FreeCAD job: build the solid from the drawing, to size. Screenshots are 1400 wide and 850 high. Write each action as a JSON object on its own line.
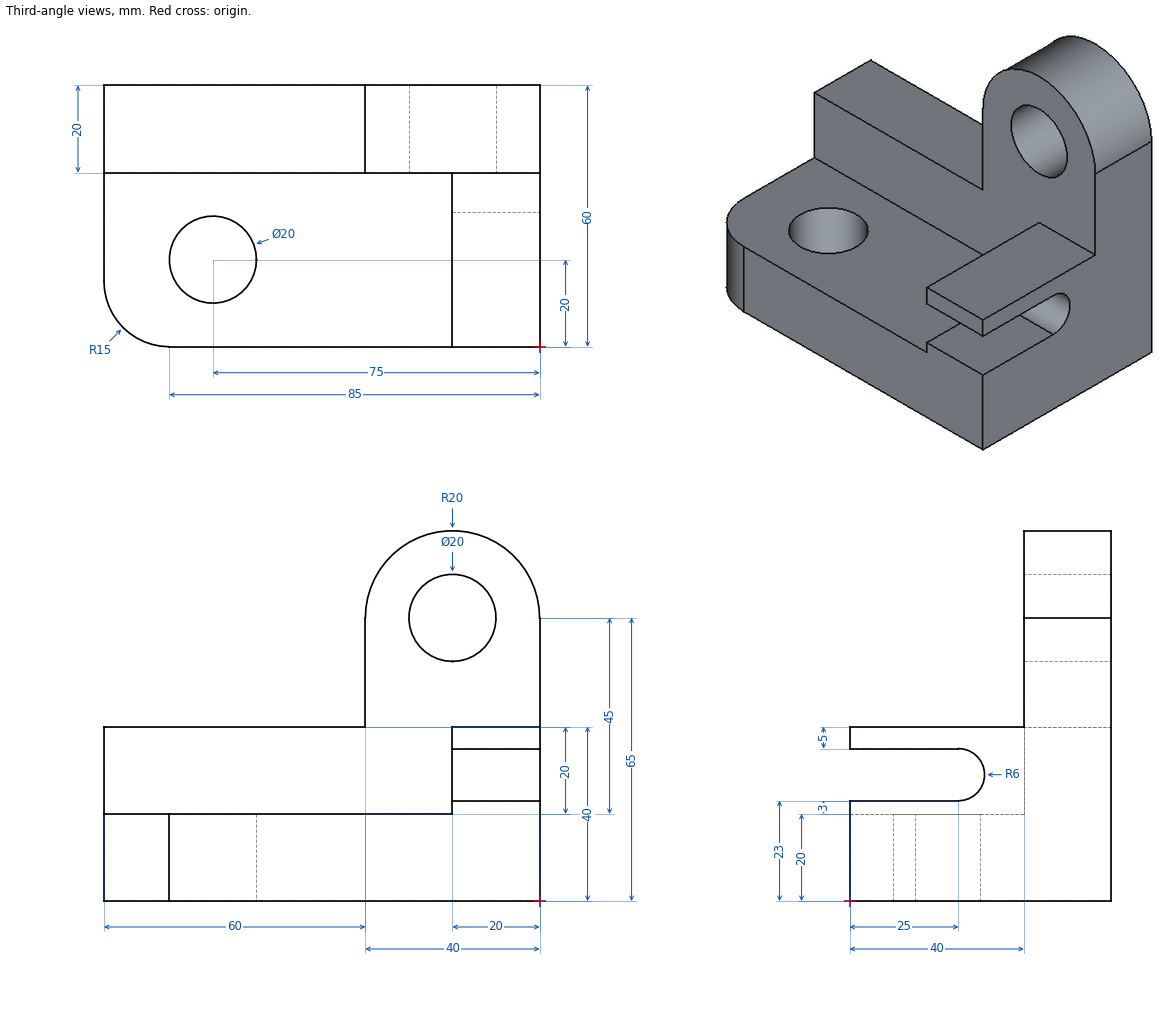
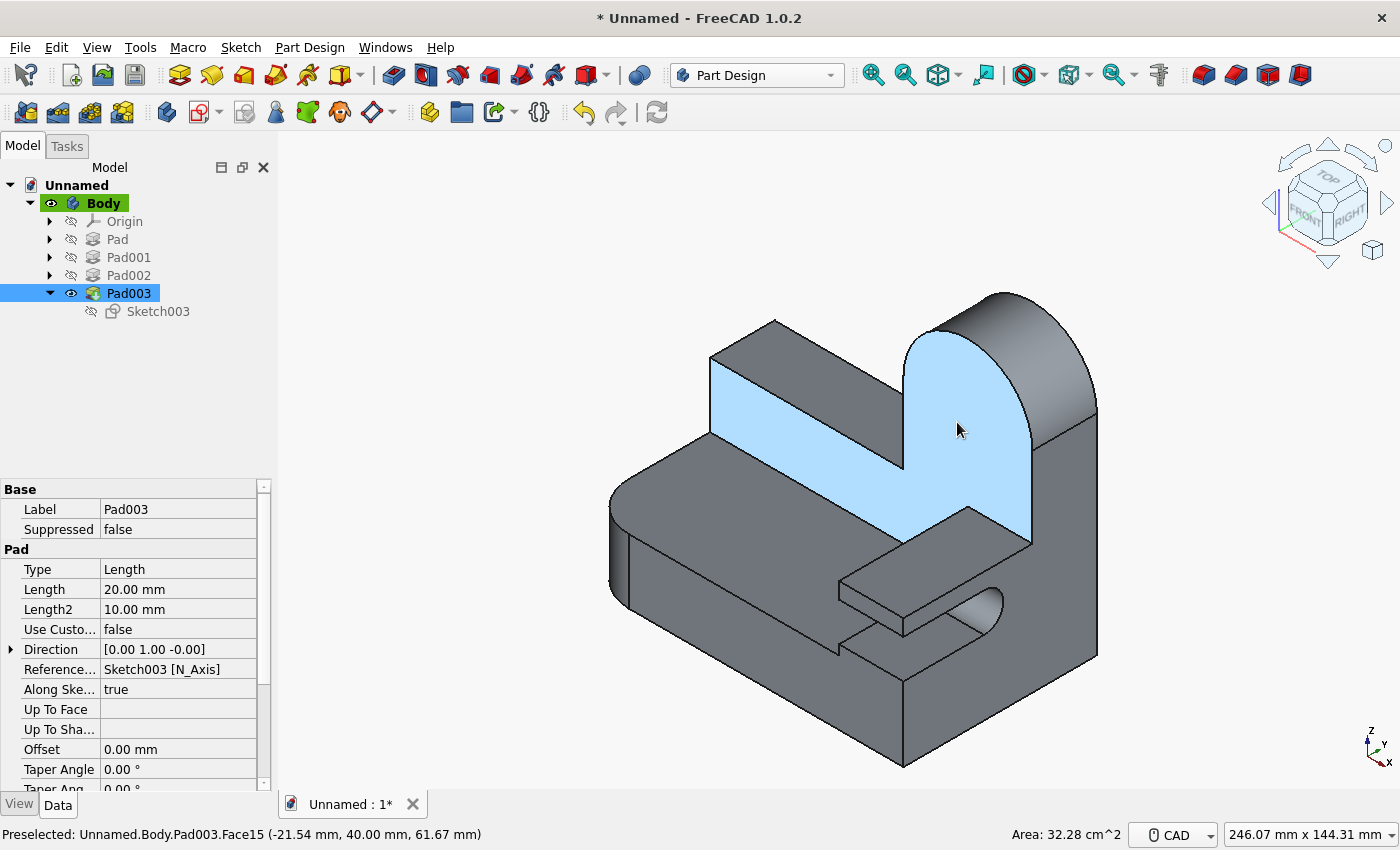
{"action": "left_click", "coordinate": [200, 112]}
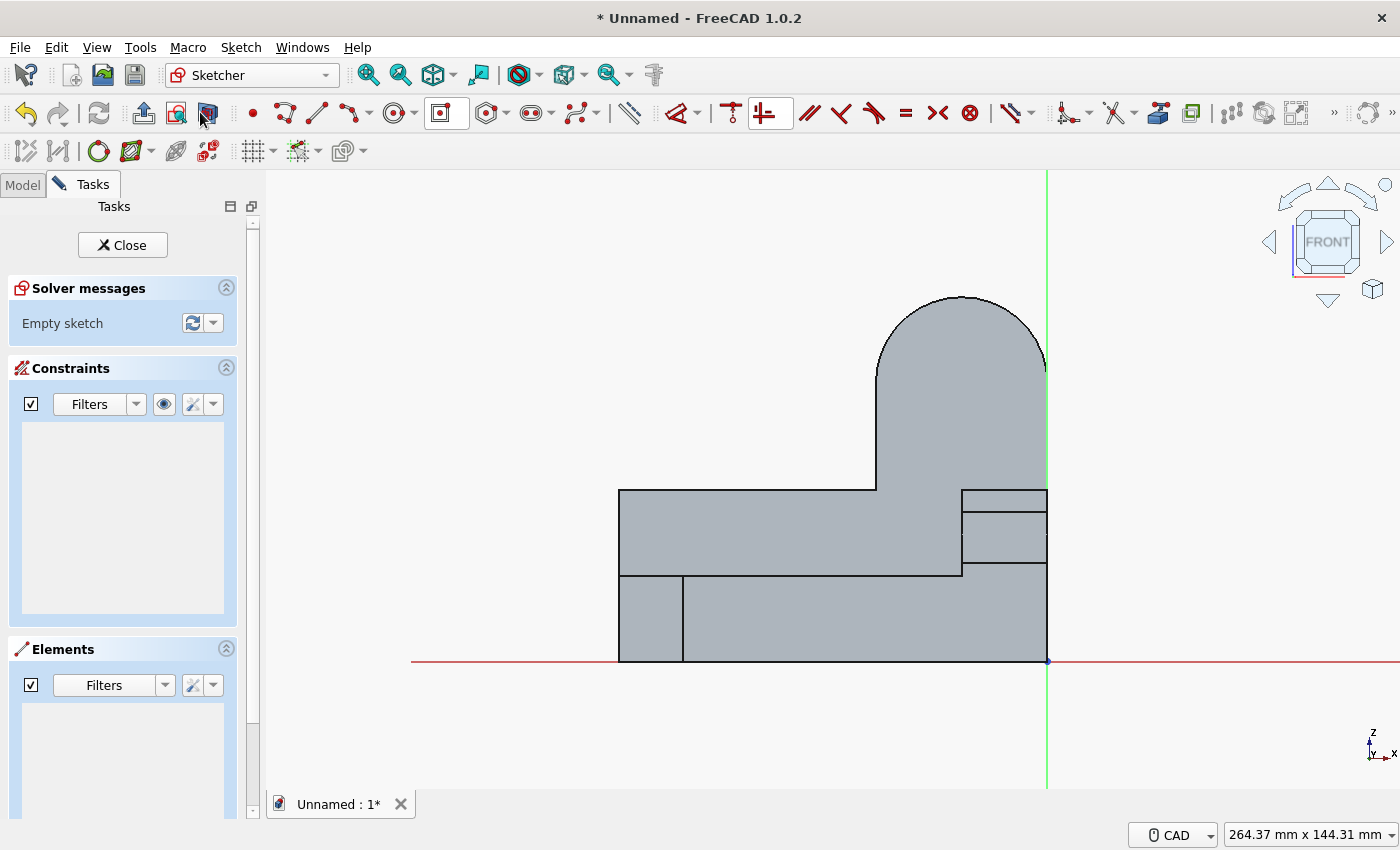
{"action": "scroll", "coordinate": [1012, 359], "scroll_direction": "up", "scroll_amount": 8}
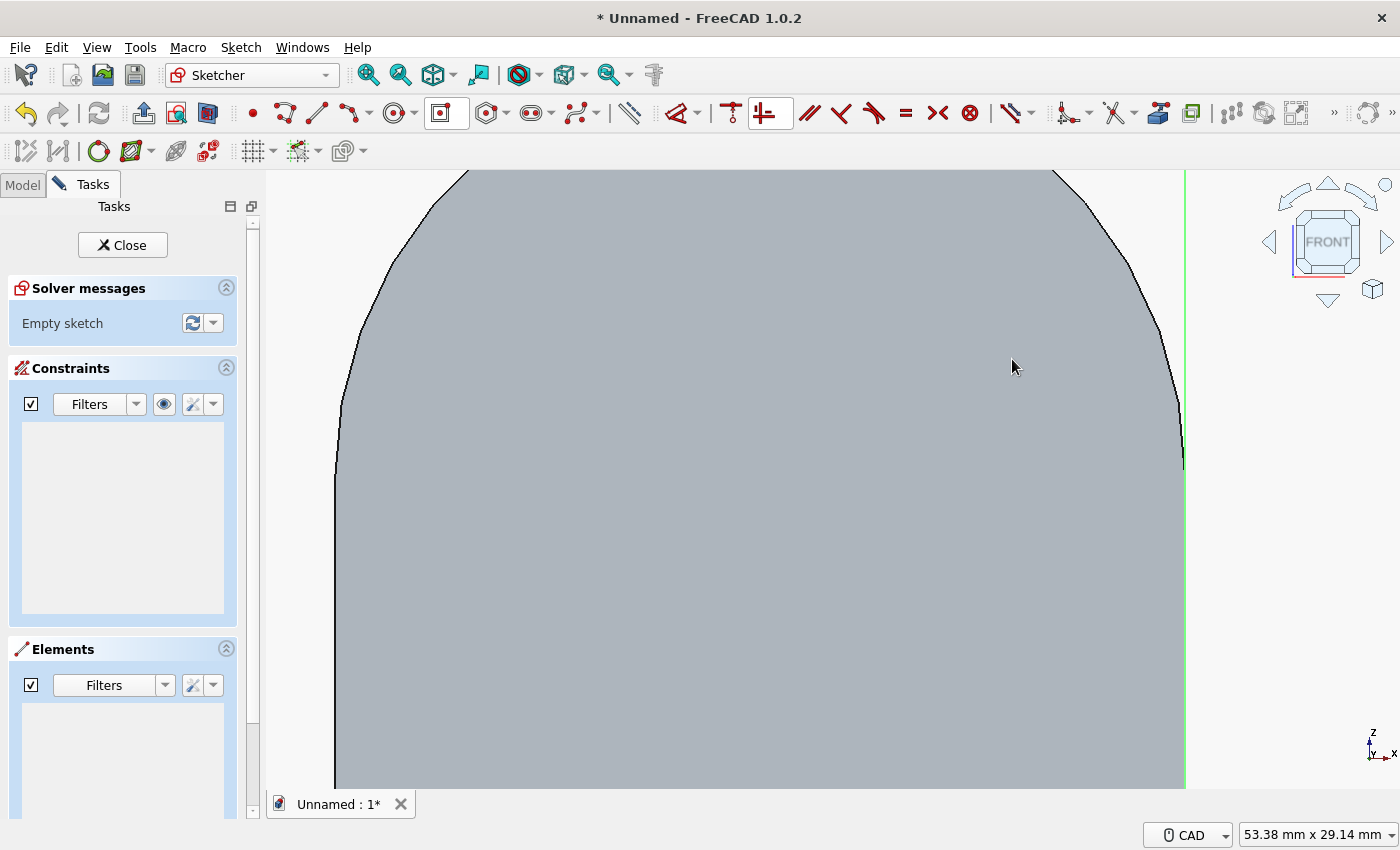
{"action": "left_click", "coordinate": [394, 114]}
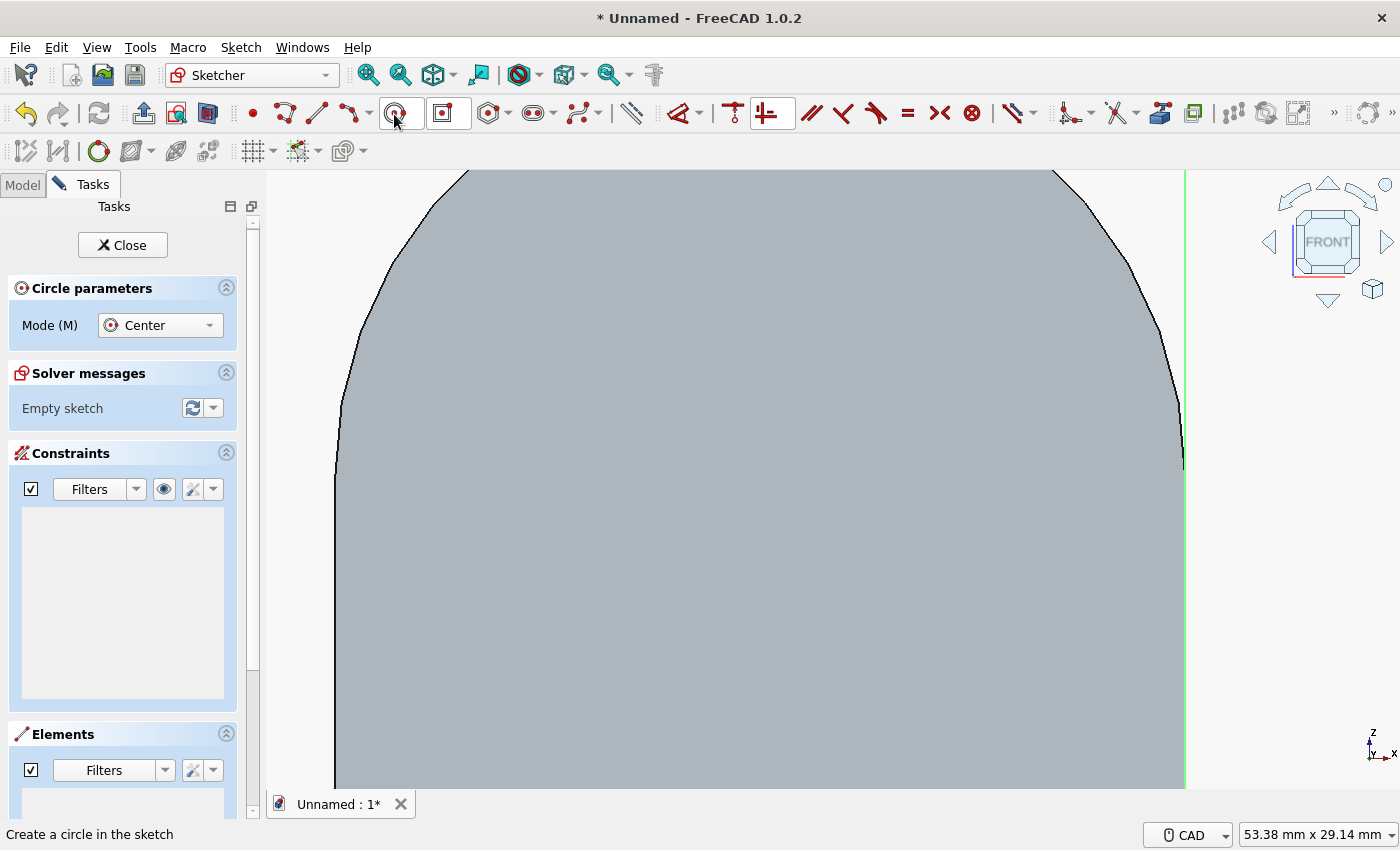
{"action": "left_click", "coordinate": [760, 477]}
{"action": "left_click", "coordinate": [910, 326]}
{"action": "key", "text": "Escape"}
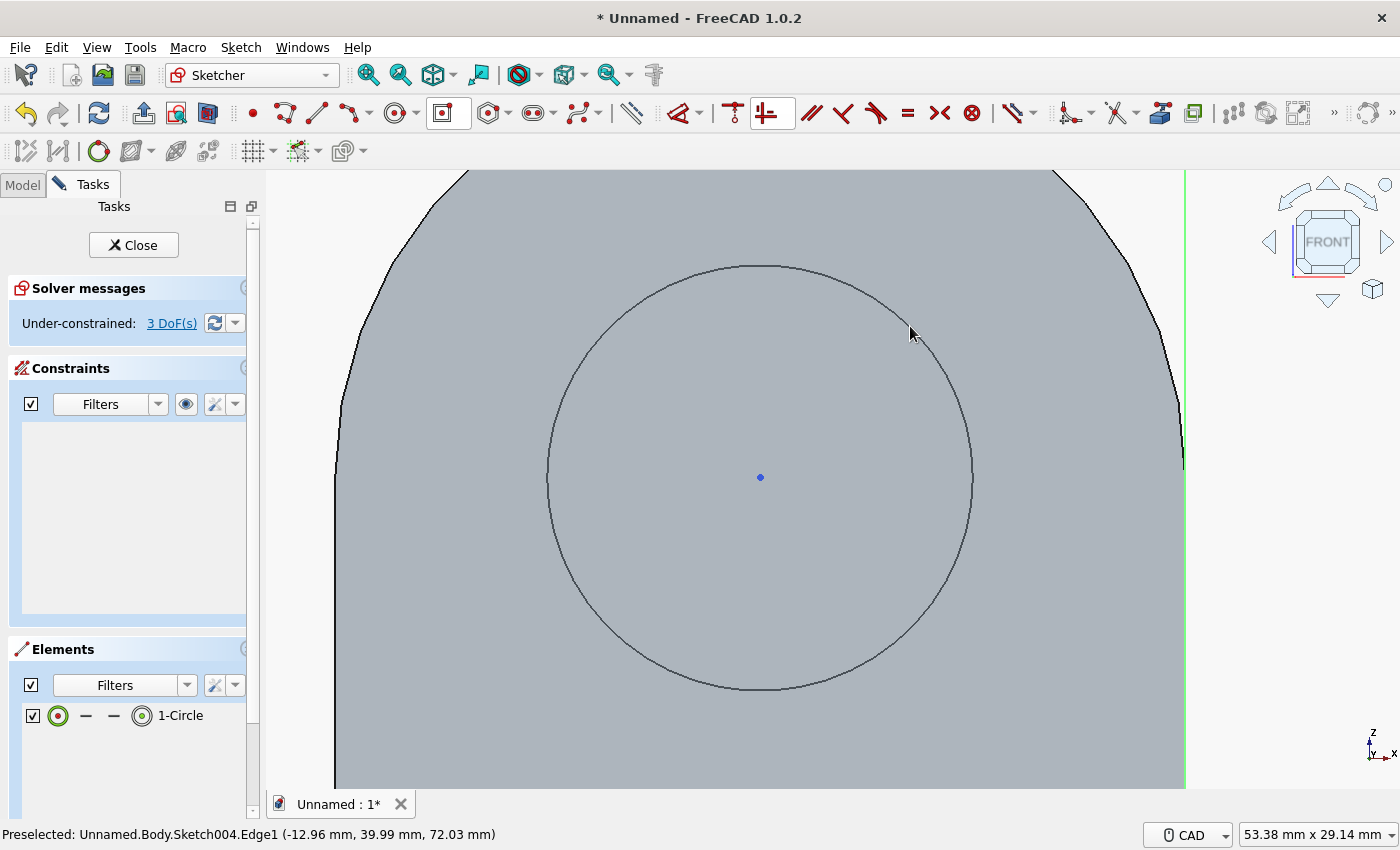
{"action": "left_click", "coordinate": [678, 114]}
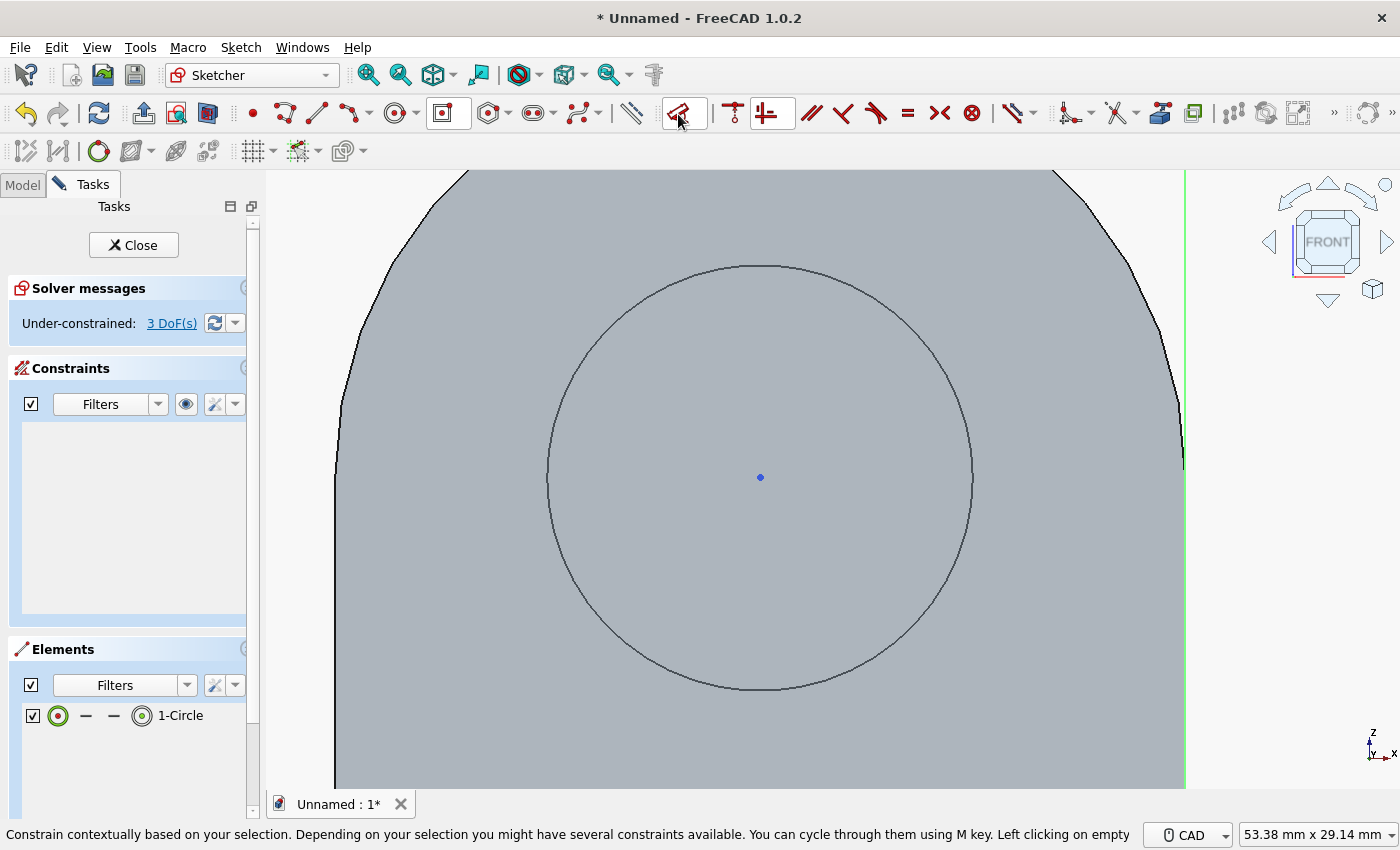
{"action": "left_click", "coordinate": [910, 327]}
{"action": "left_click", "coordinate": [933, 304]}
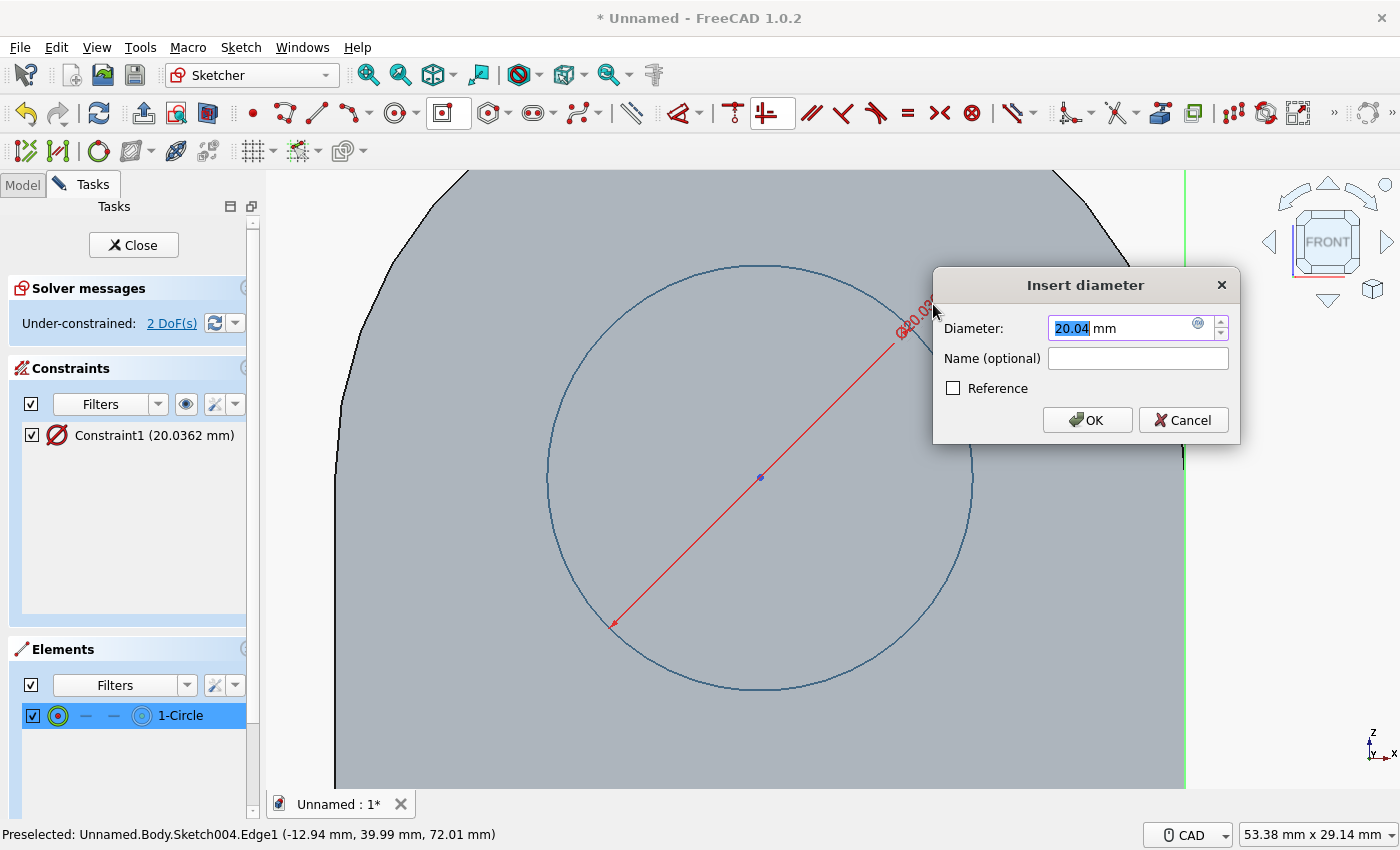
{"action": "type", "text": "20"}
{"action": "key", "text": "Return"}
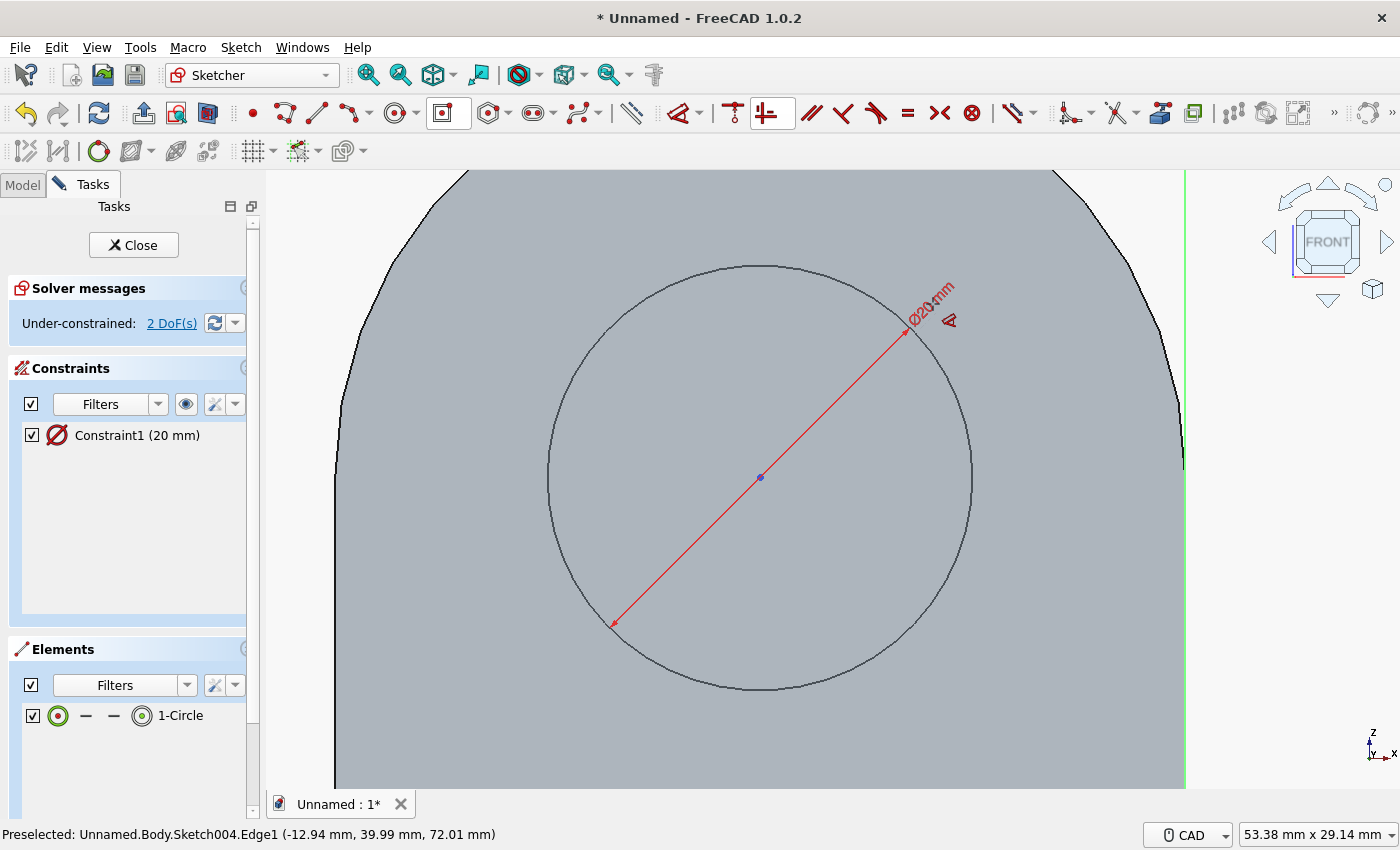
{"action": "left_click", "coordinate": [760, 478]}
{"action": "left_click", "coordinate": [875, 444]}